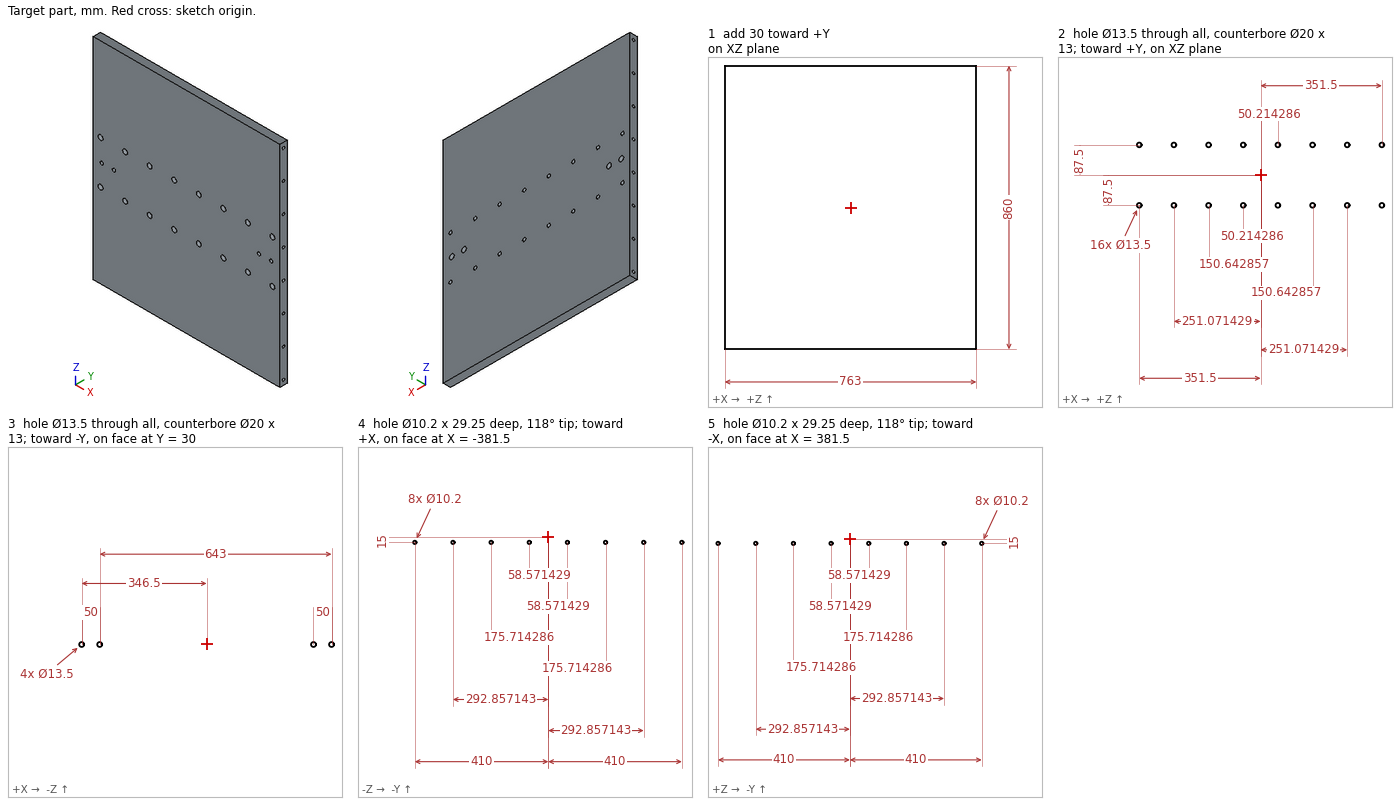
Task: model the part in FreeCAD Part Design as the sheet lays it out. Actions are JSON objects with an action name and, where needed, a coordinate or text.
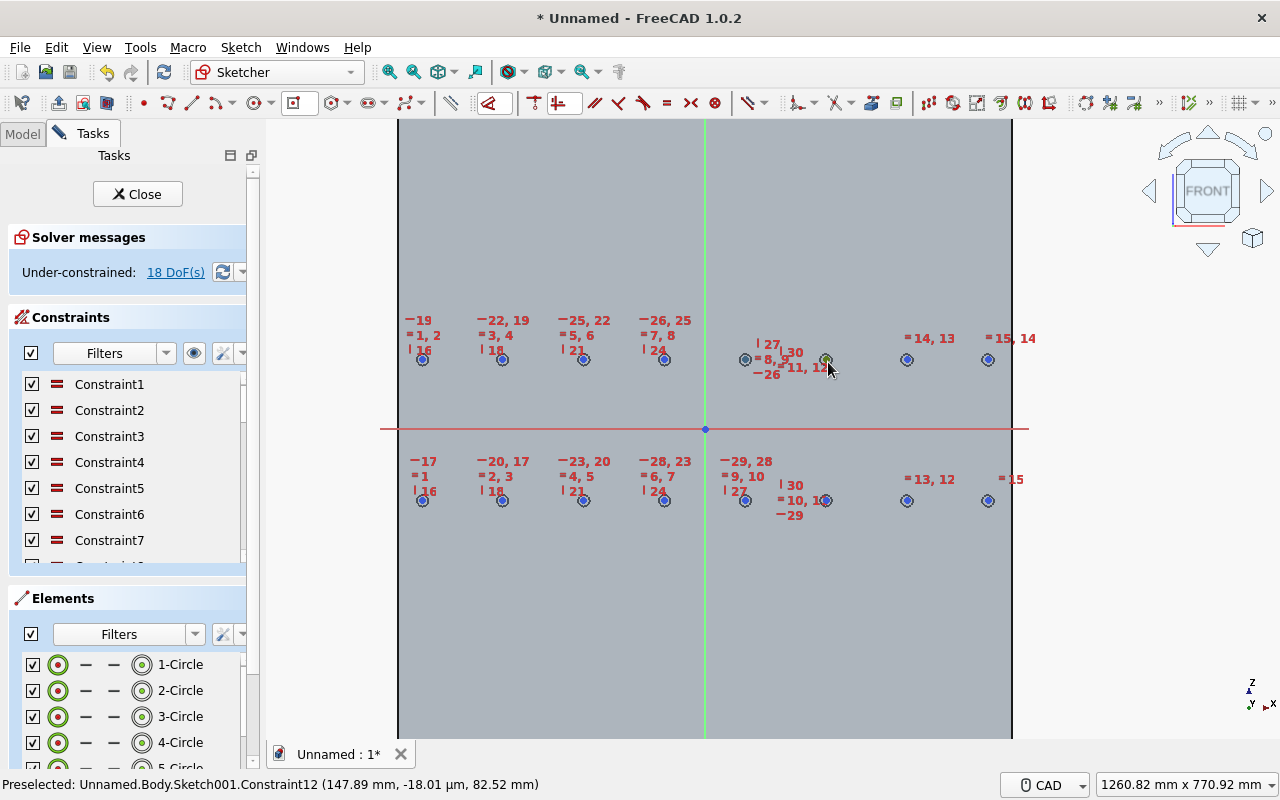
{"action": "key", "text": "h"}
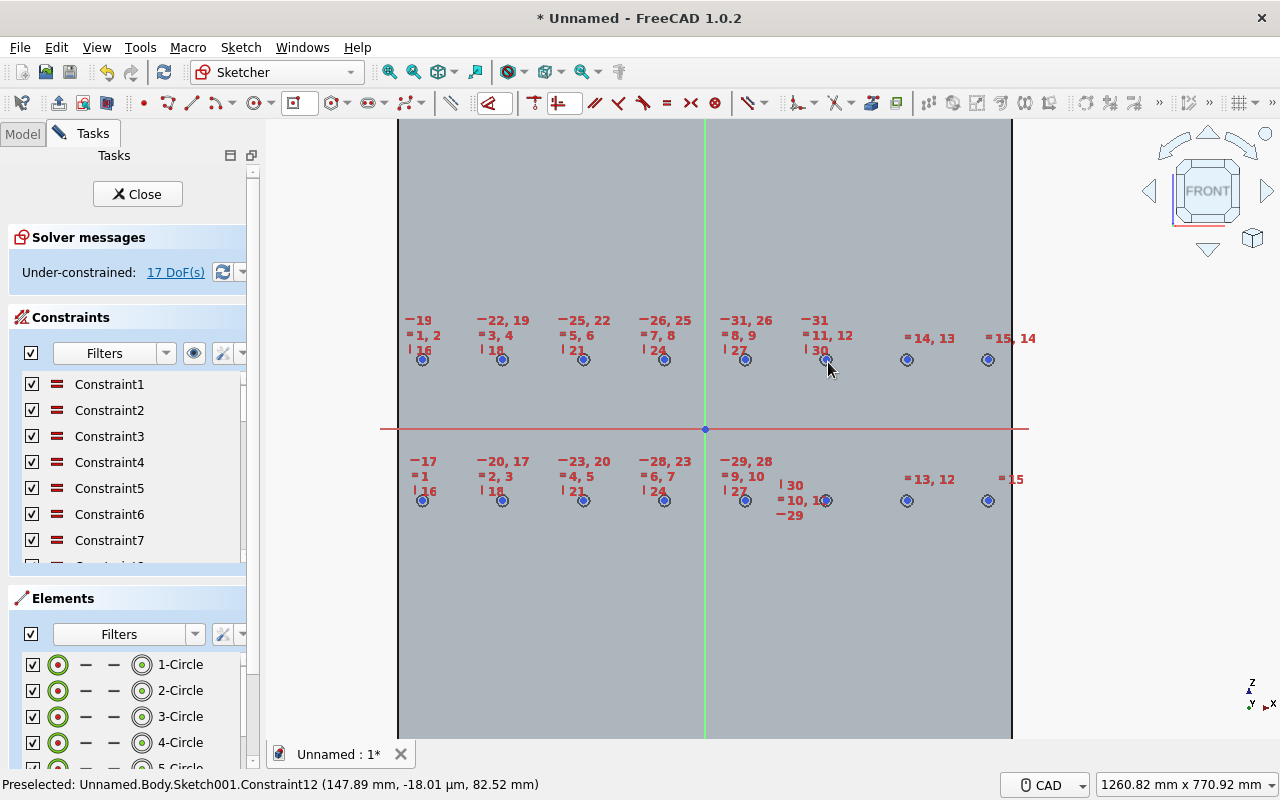
{"action": "left_click", "coordinate": [826, 501]}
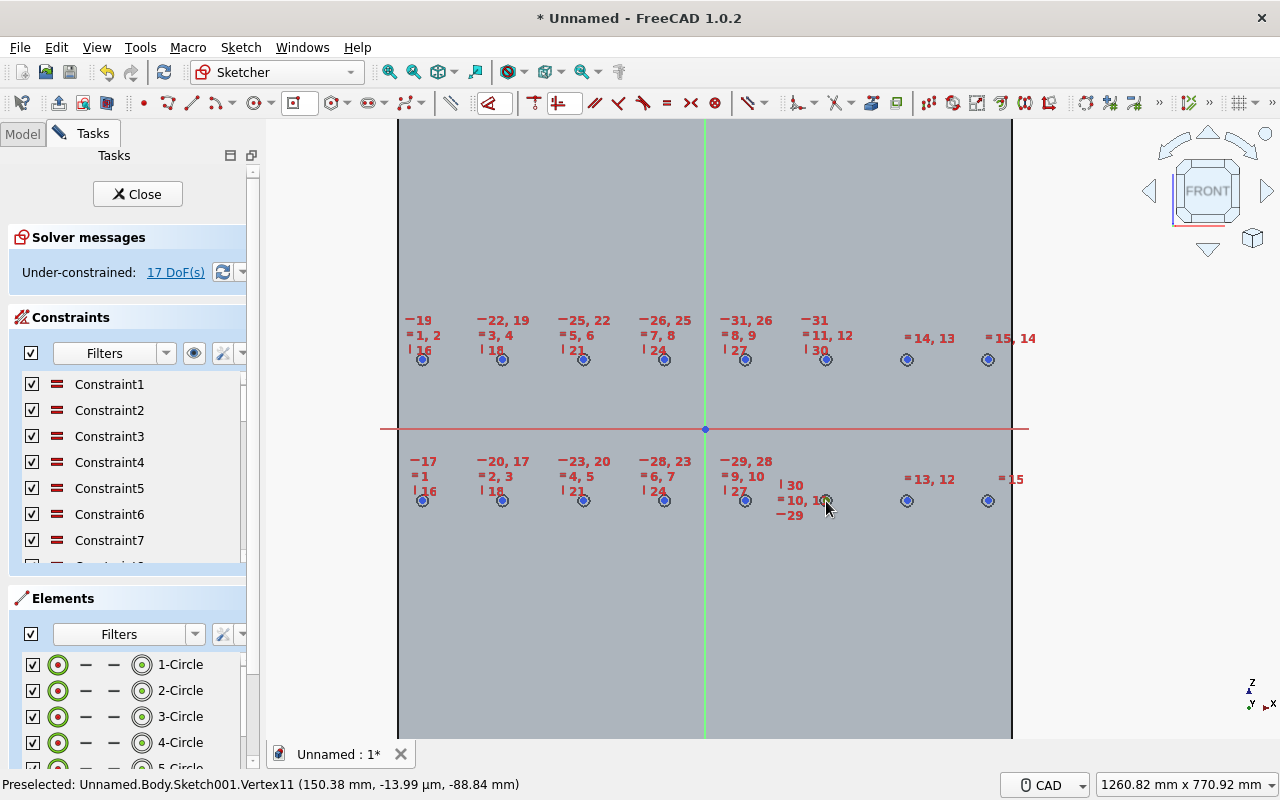
{"action": "left_click", "coordinate": [907, 501]}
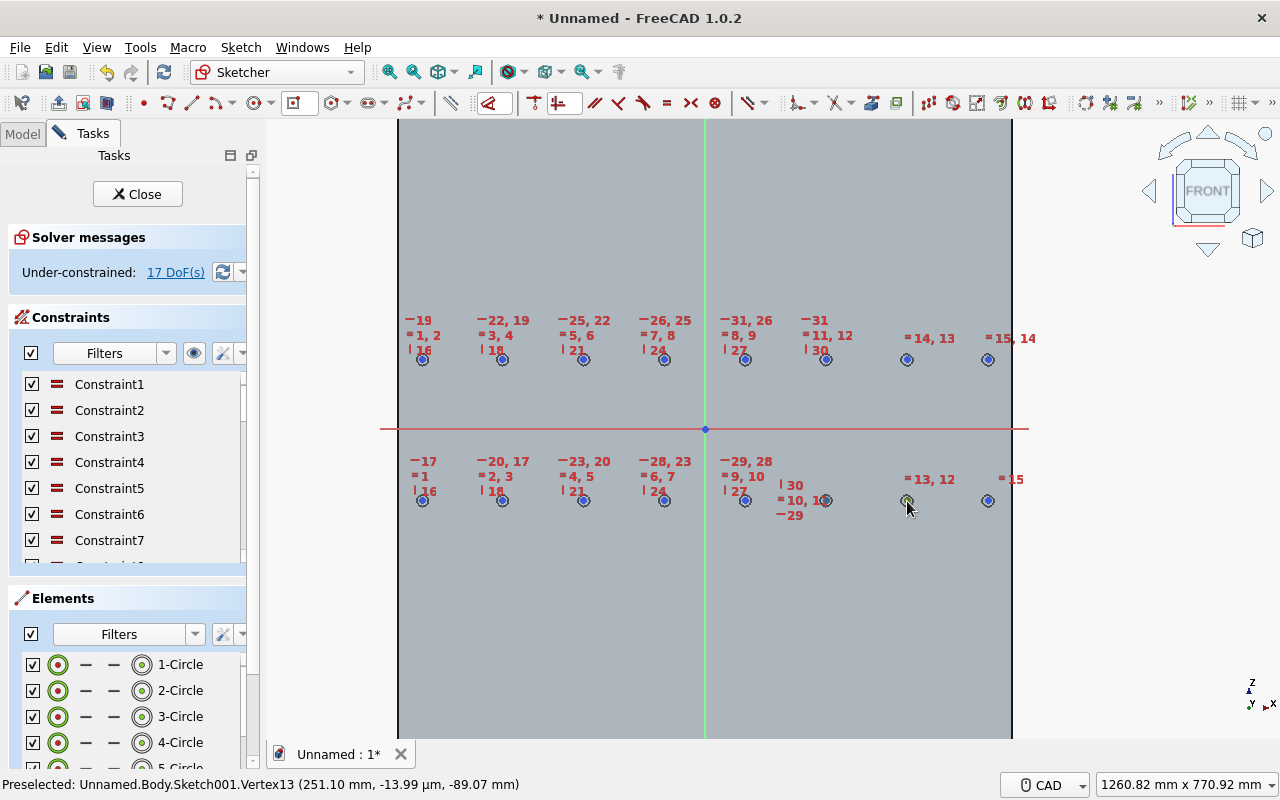
{"action": "key", "text": "h"}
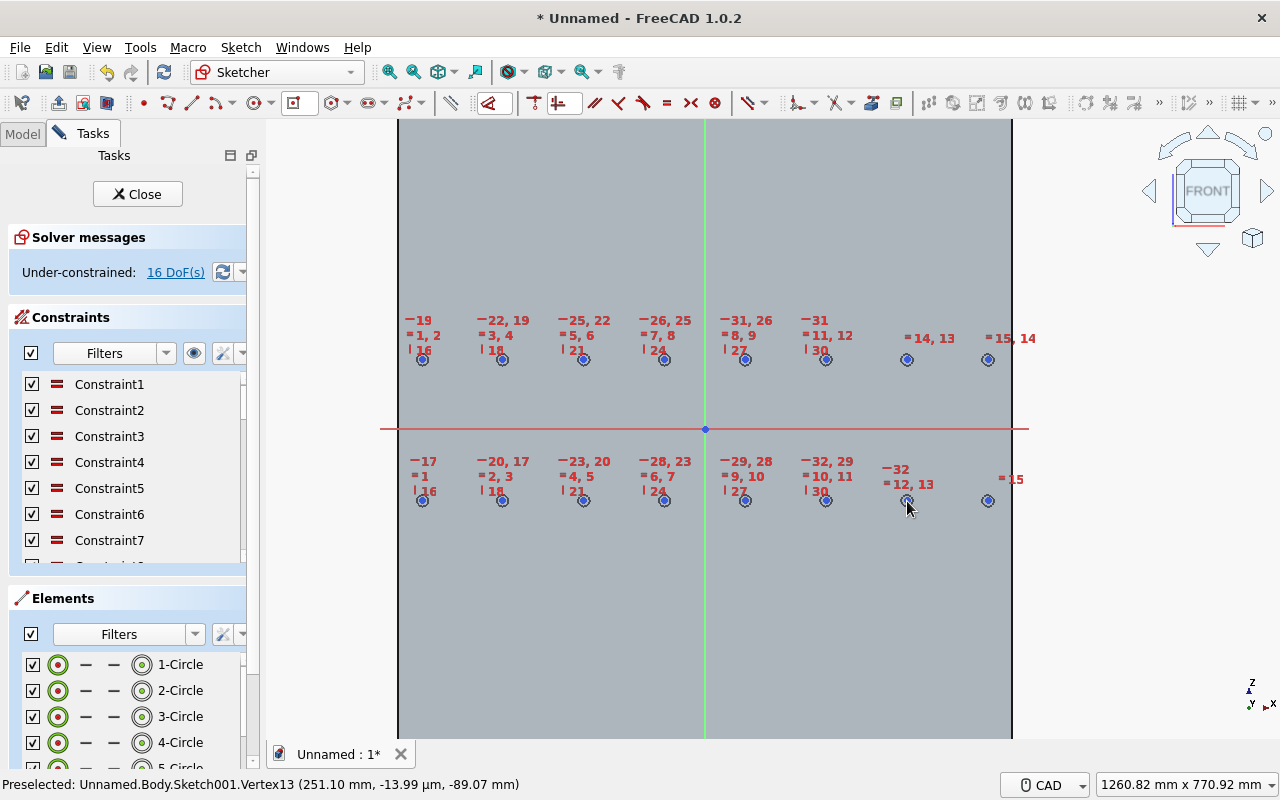
{"action": "left_click", "coordinate": [907, 501]}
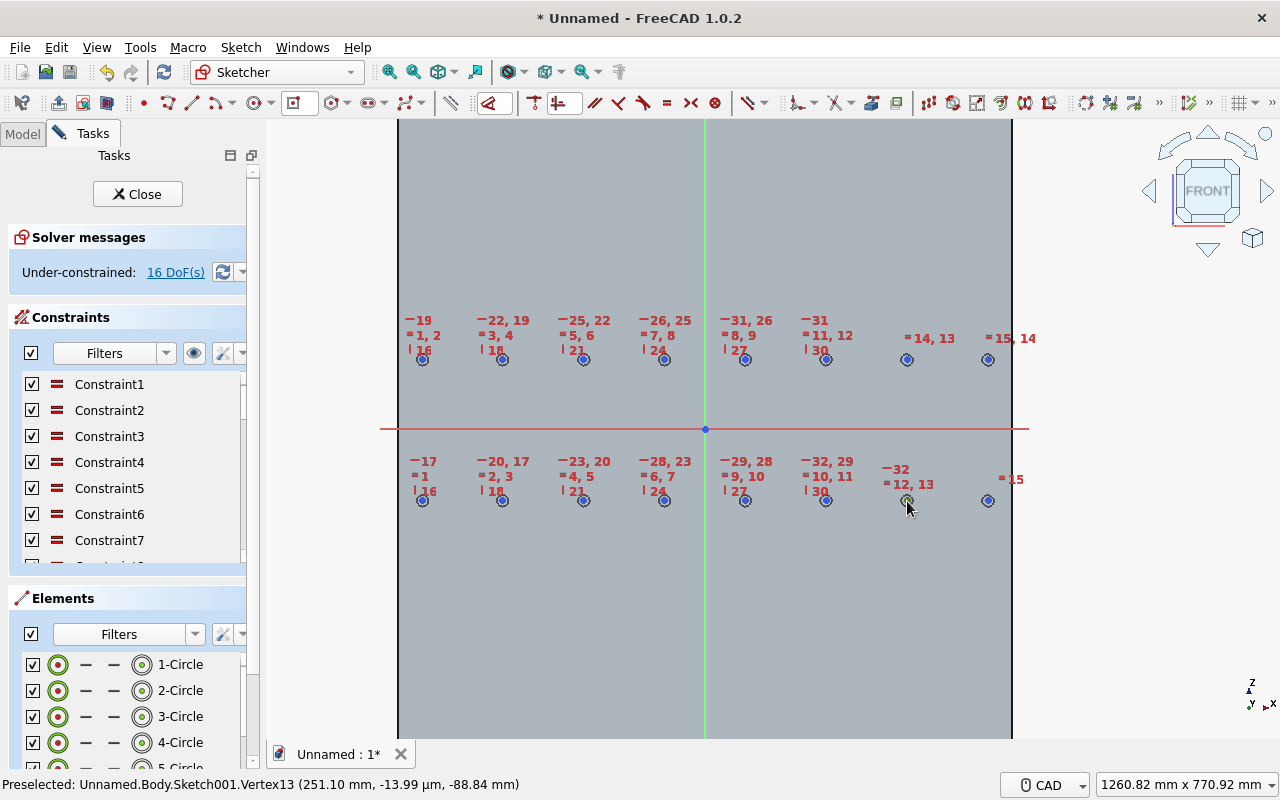
{"action": "left_click", "coordinate": [907, 360]}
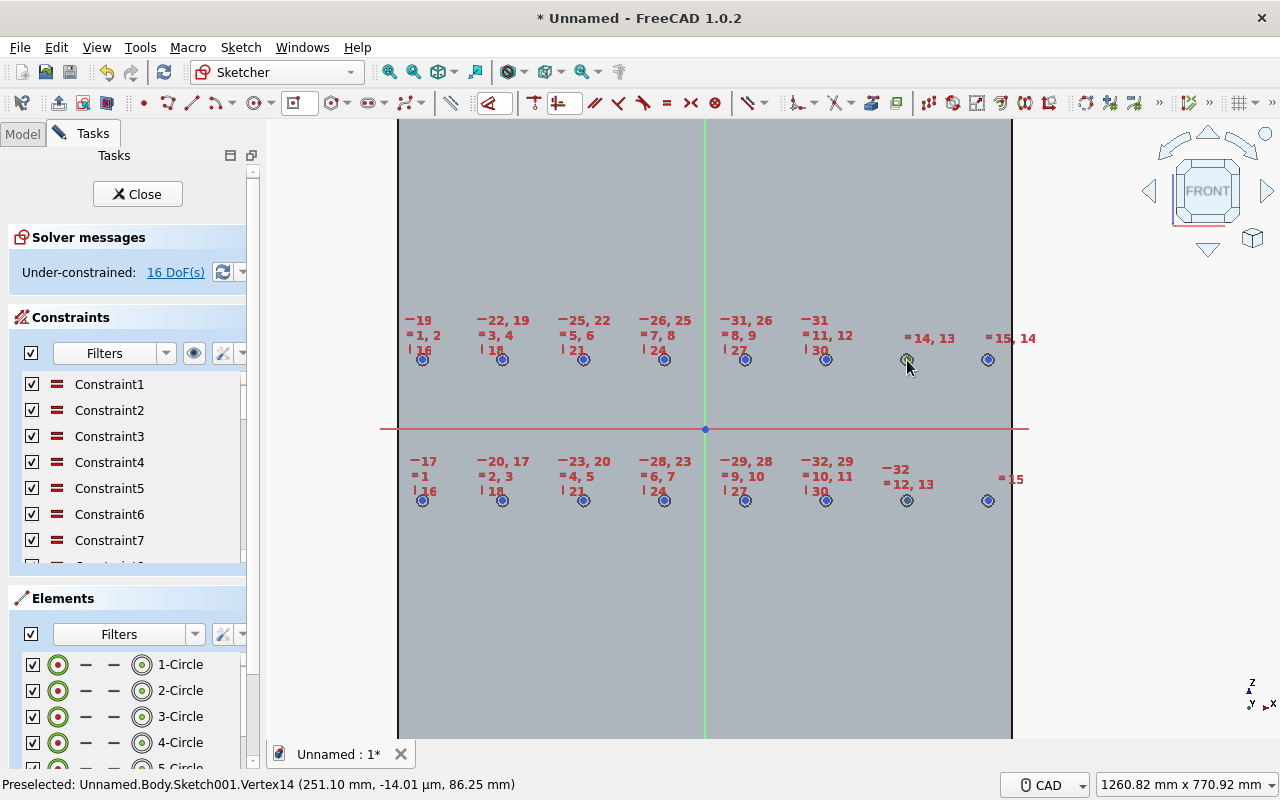
{"action": "key", "text": "v"}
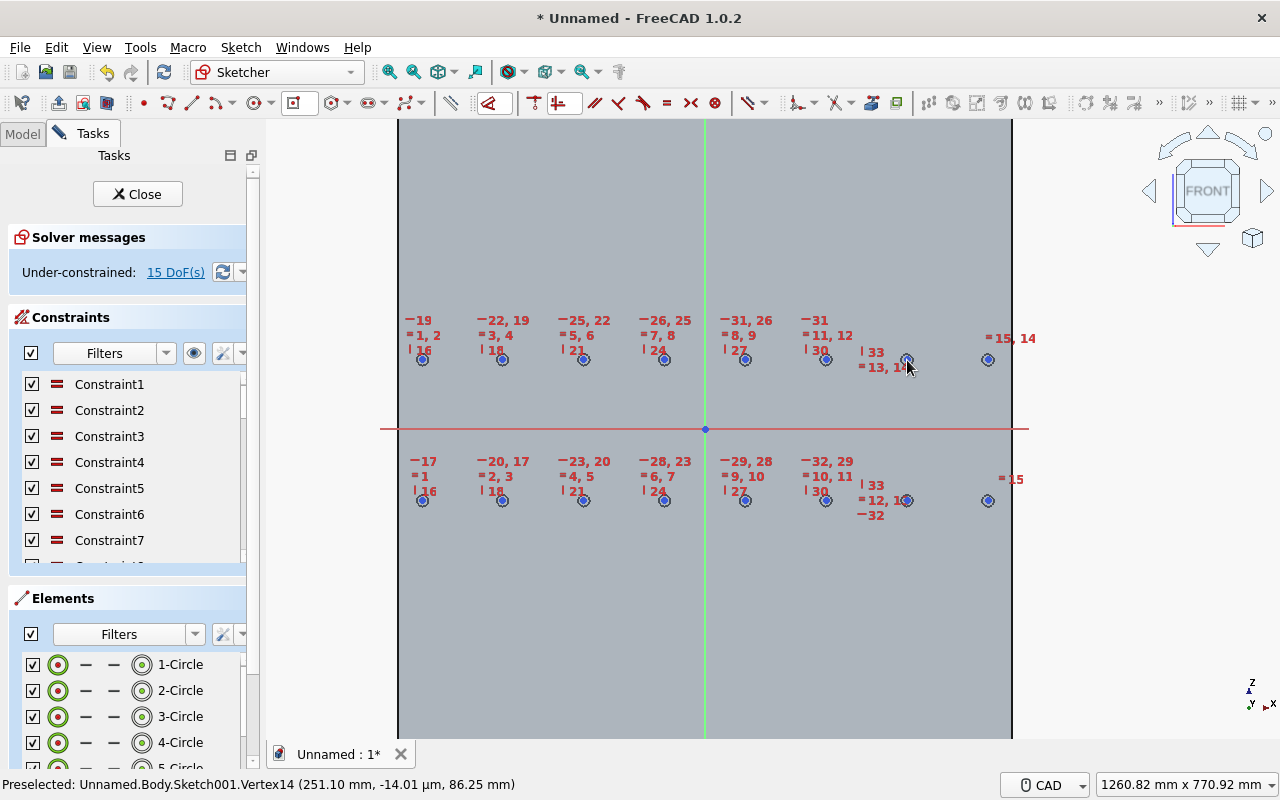
{"action": "left_click", "coordinate": [826, 360]}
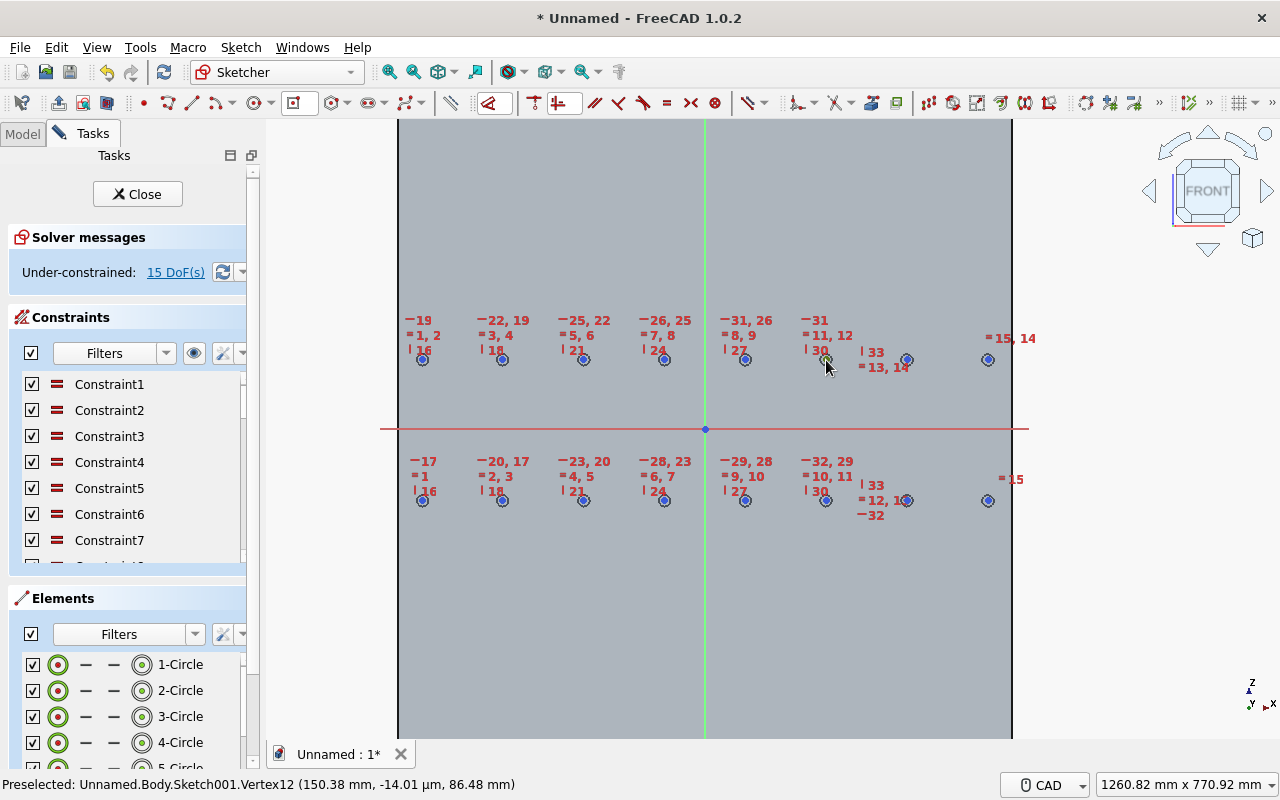
{"action": "left_click", "coordinate": [909, 362]}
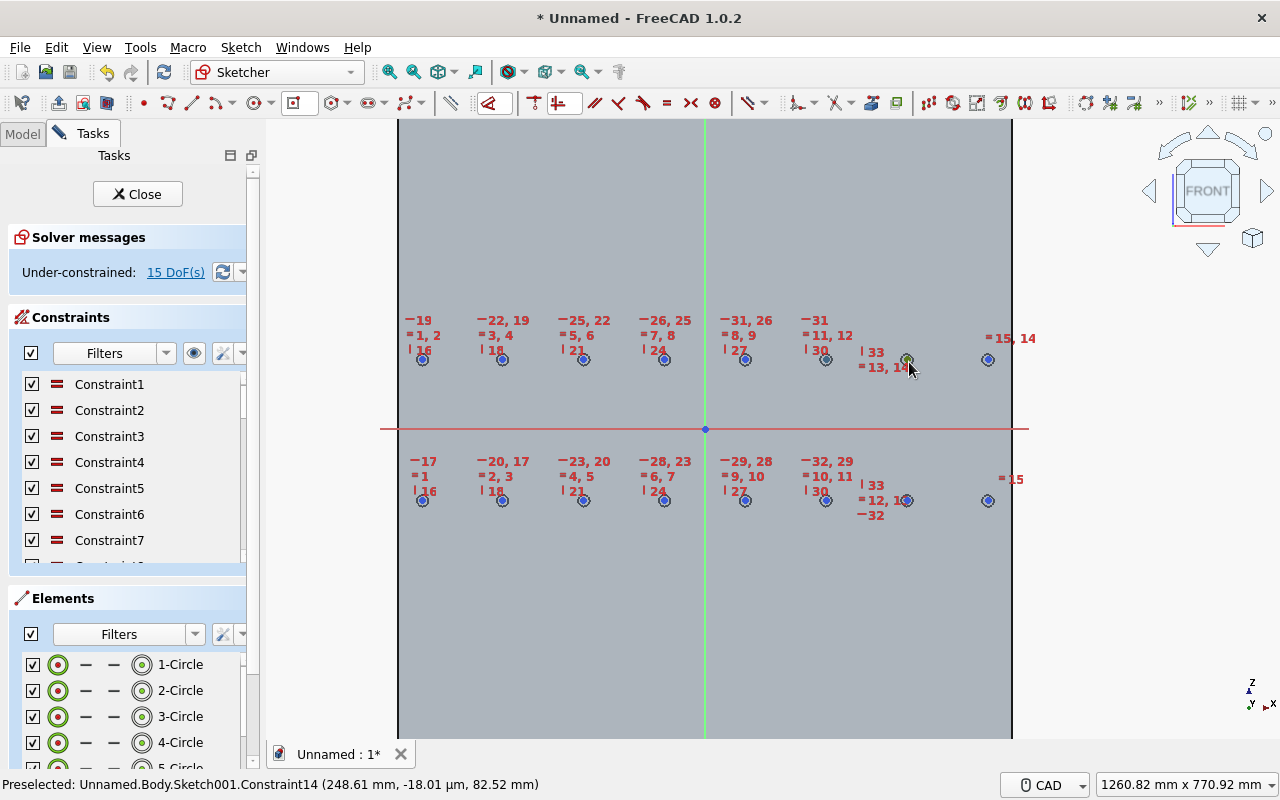
{"action": "left_click", "coordinate": [576, 104]}